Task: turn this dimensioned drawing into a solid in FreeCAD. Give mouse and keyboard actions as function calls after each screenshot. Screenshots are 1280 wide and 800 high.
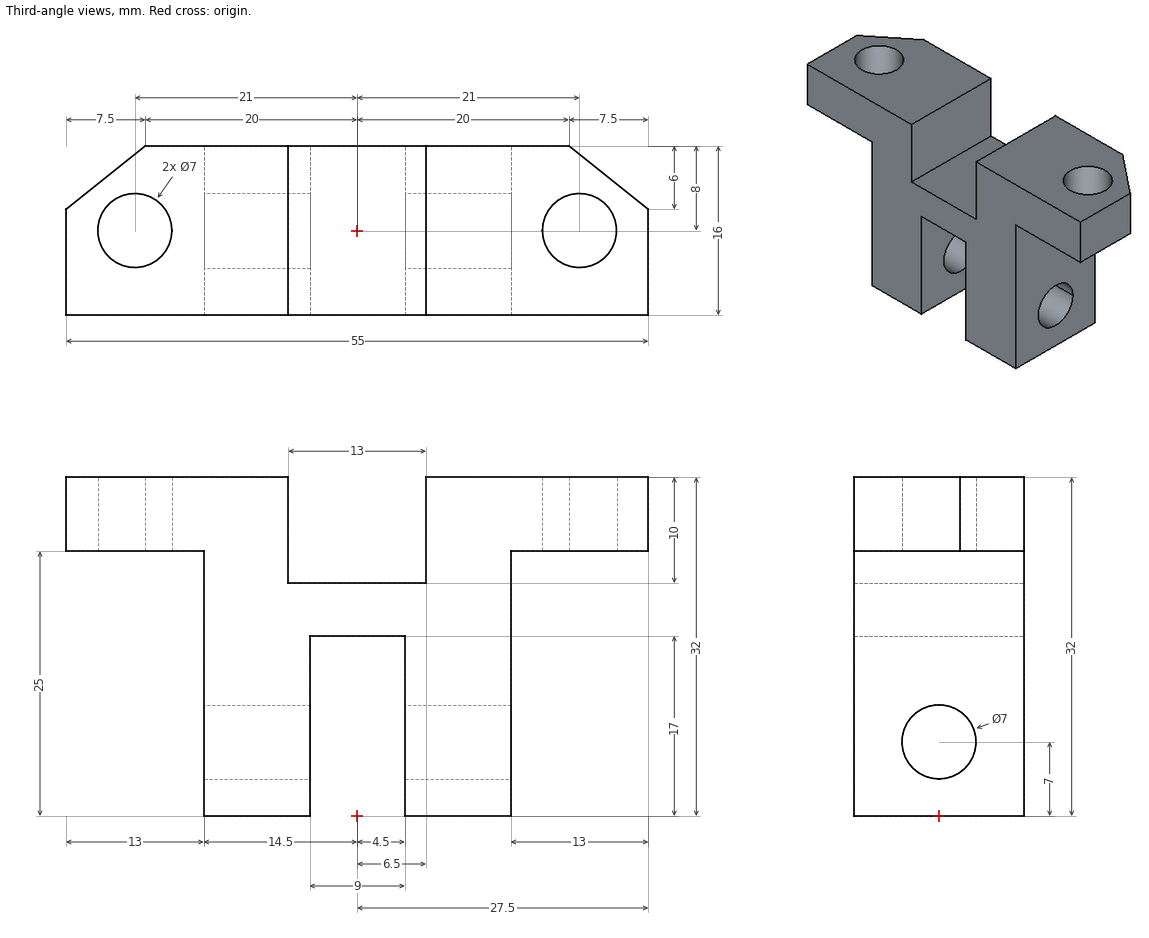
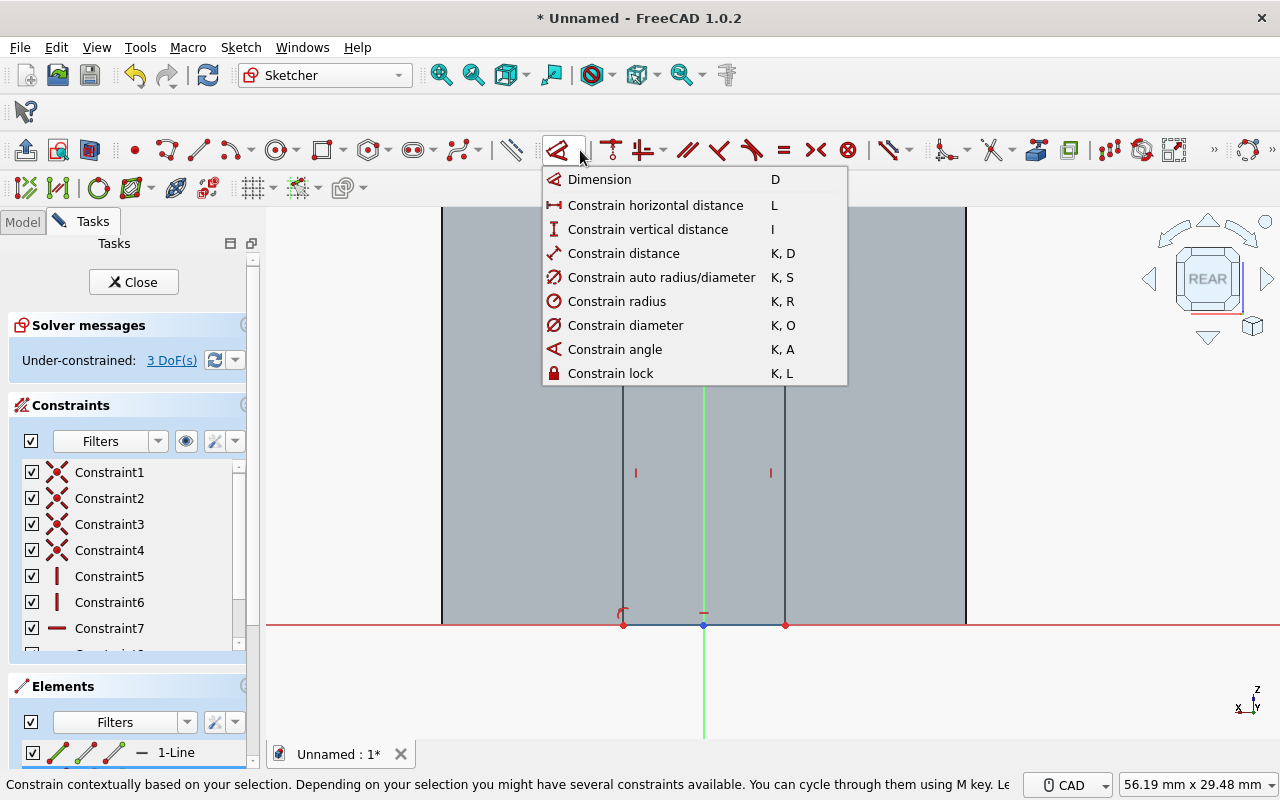
click(695, 205)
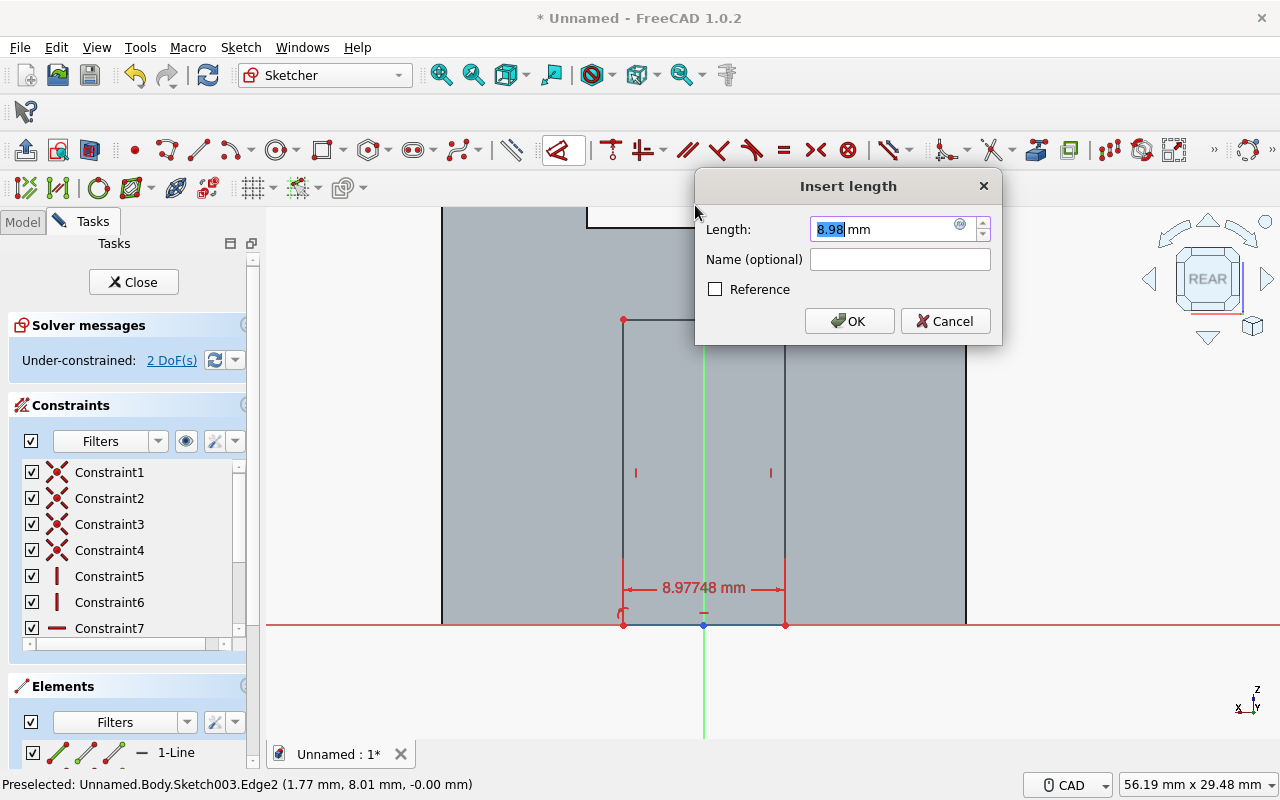
text(9)
key(Return)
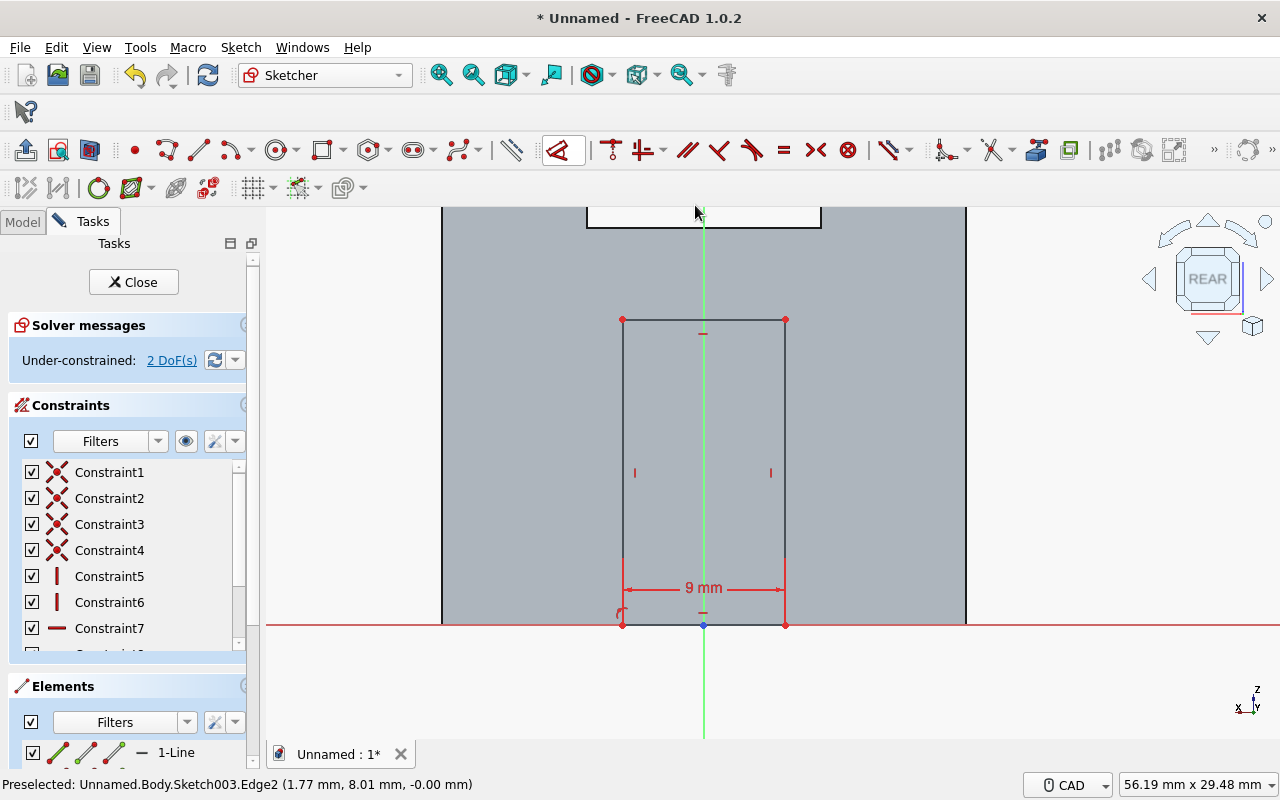
click(623, 412)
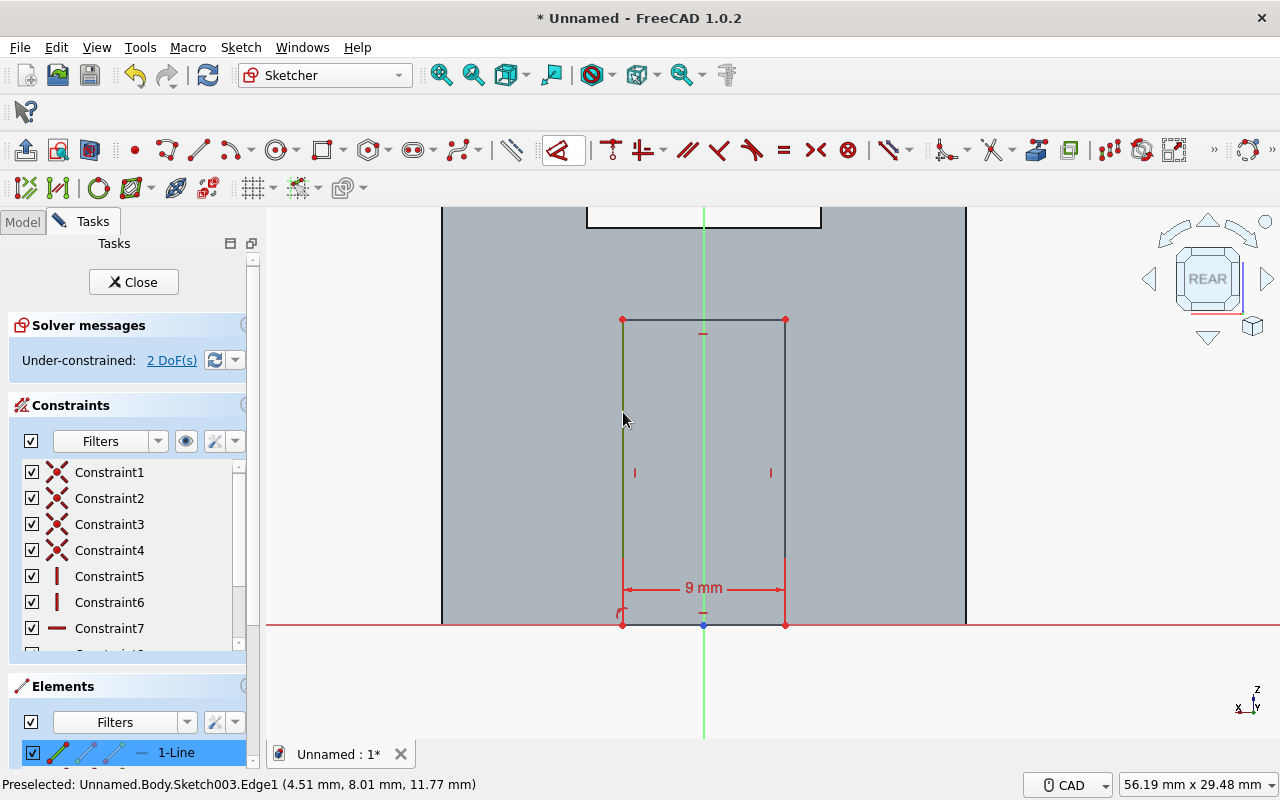
key(i)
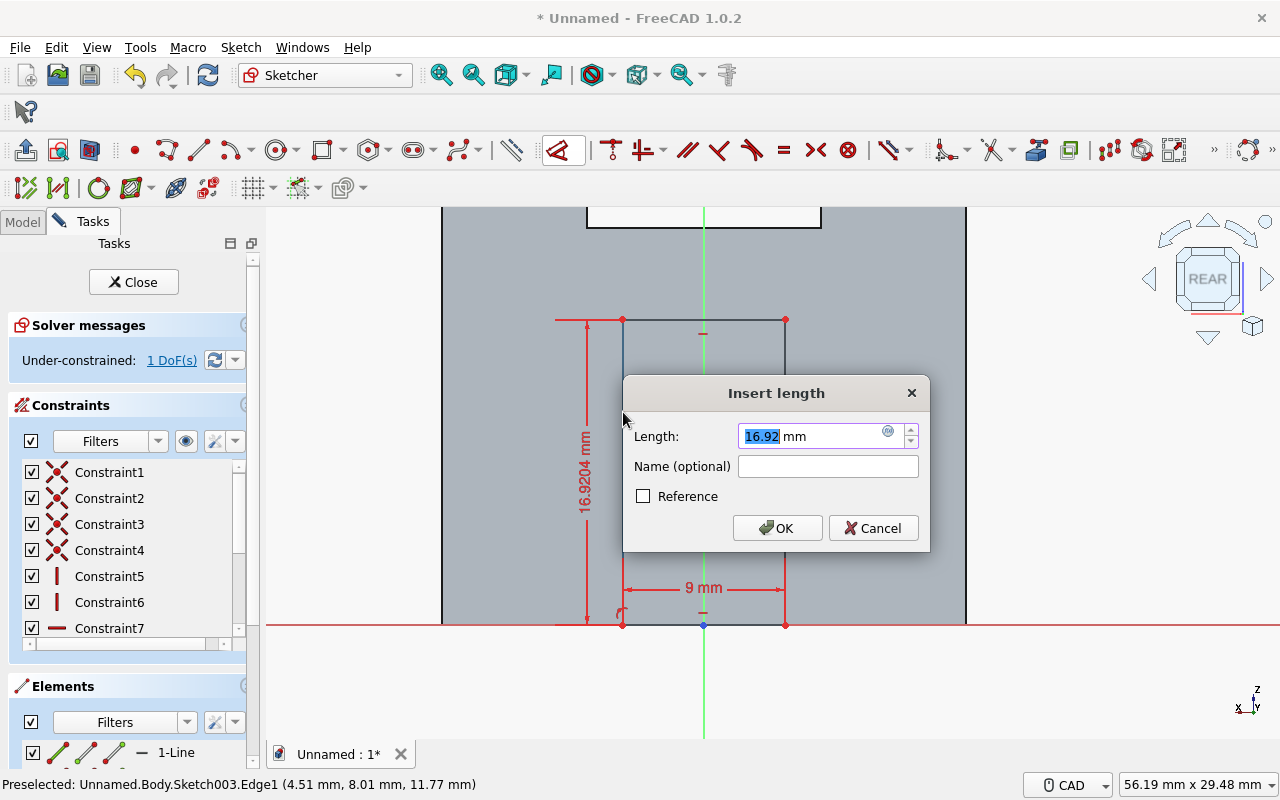
text(17)
key(Return)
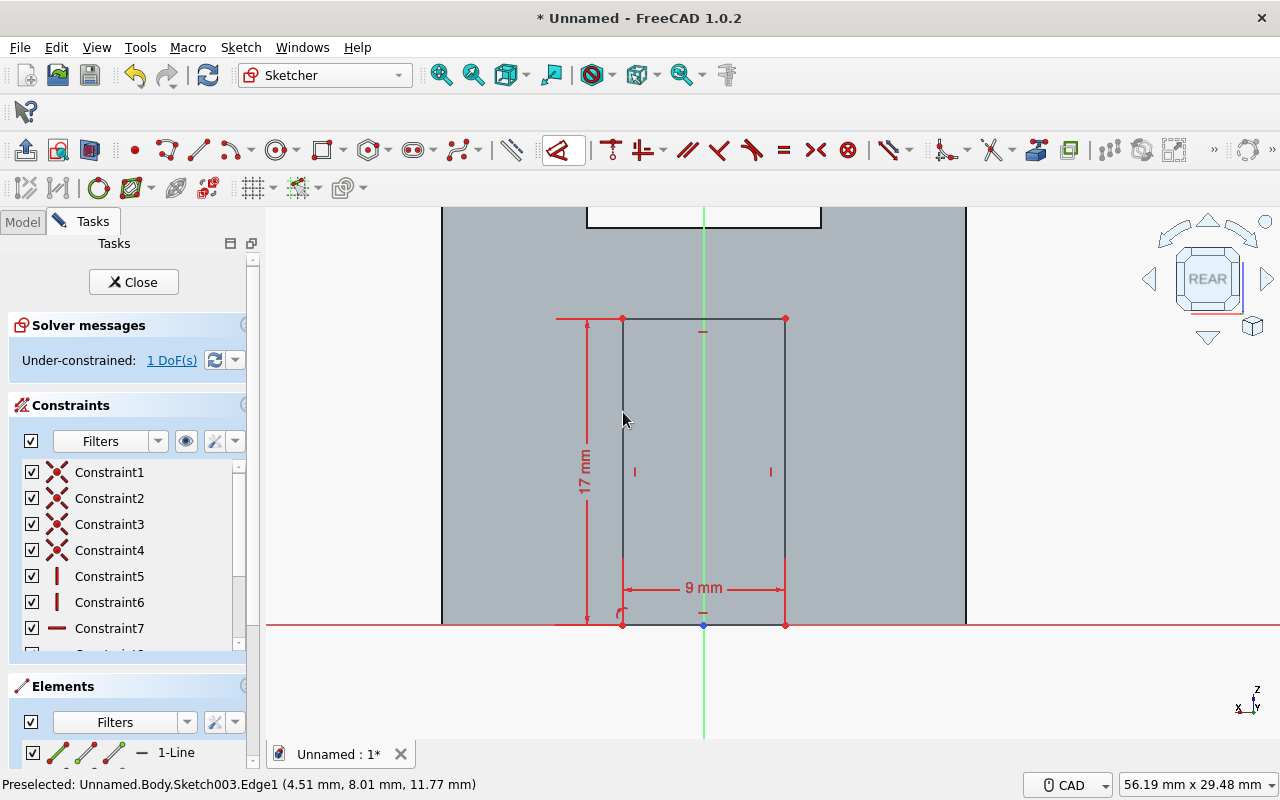
click(623, 319)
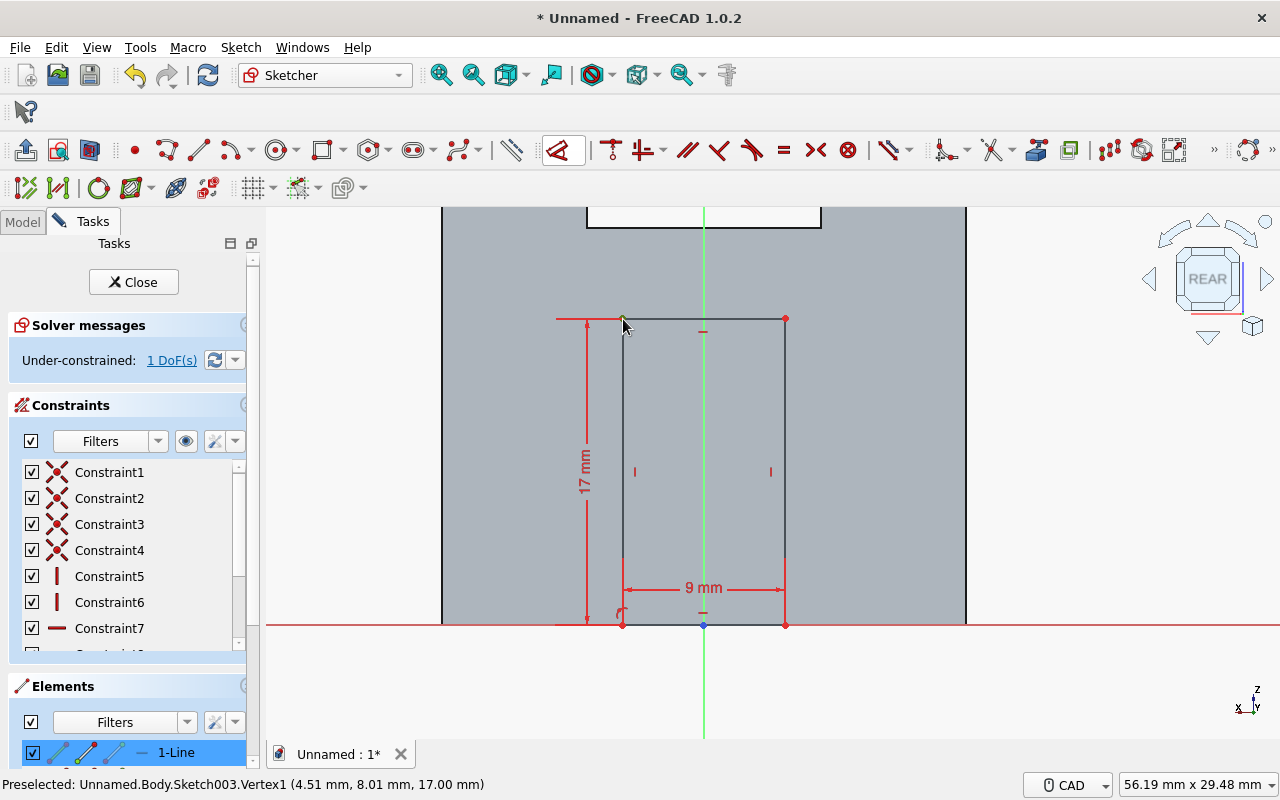
key(l)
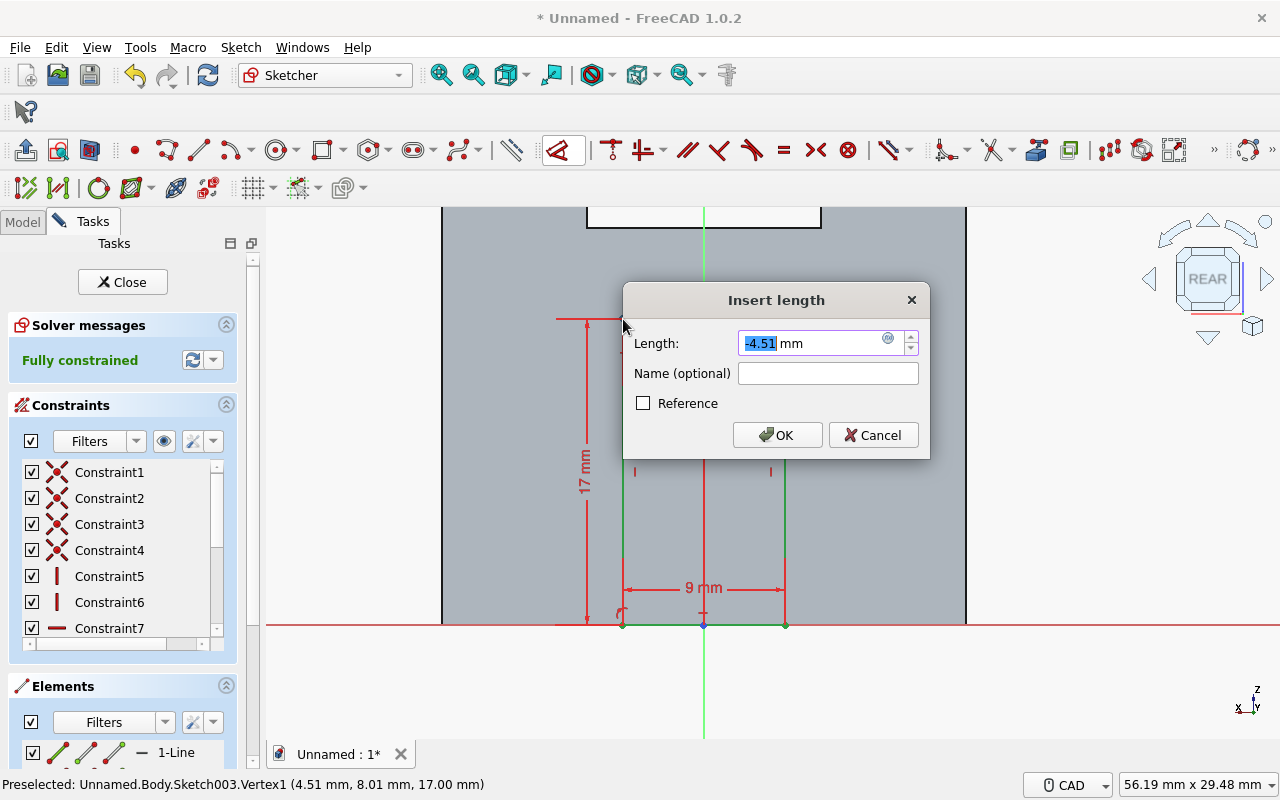
text(-4.5)
key(Return)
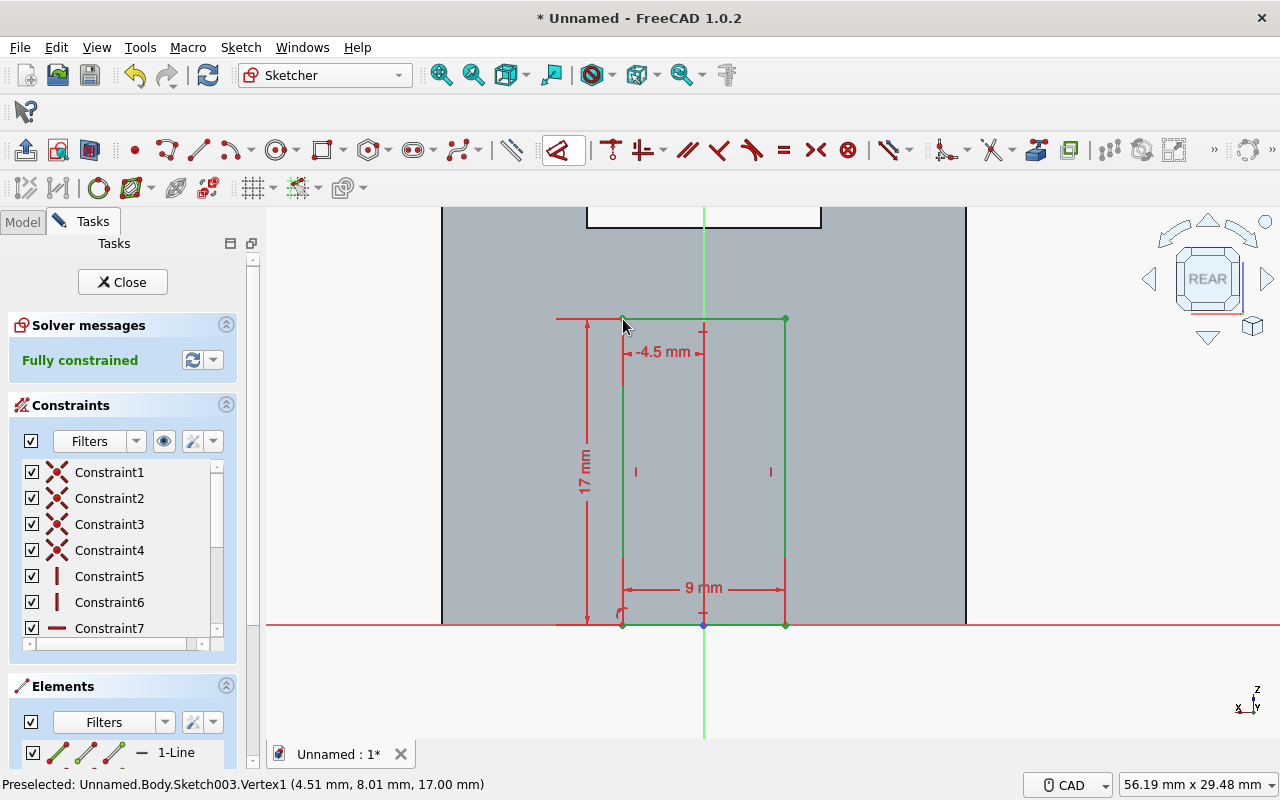
click(123, 282)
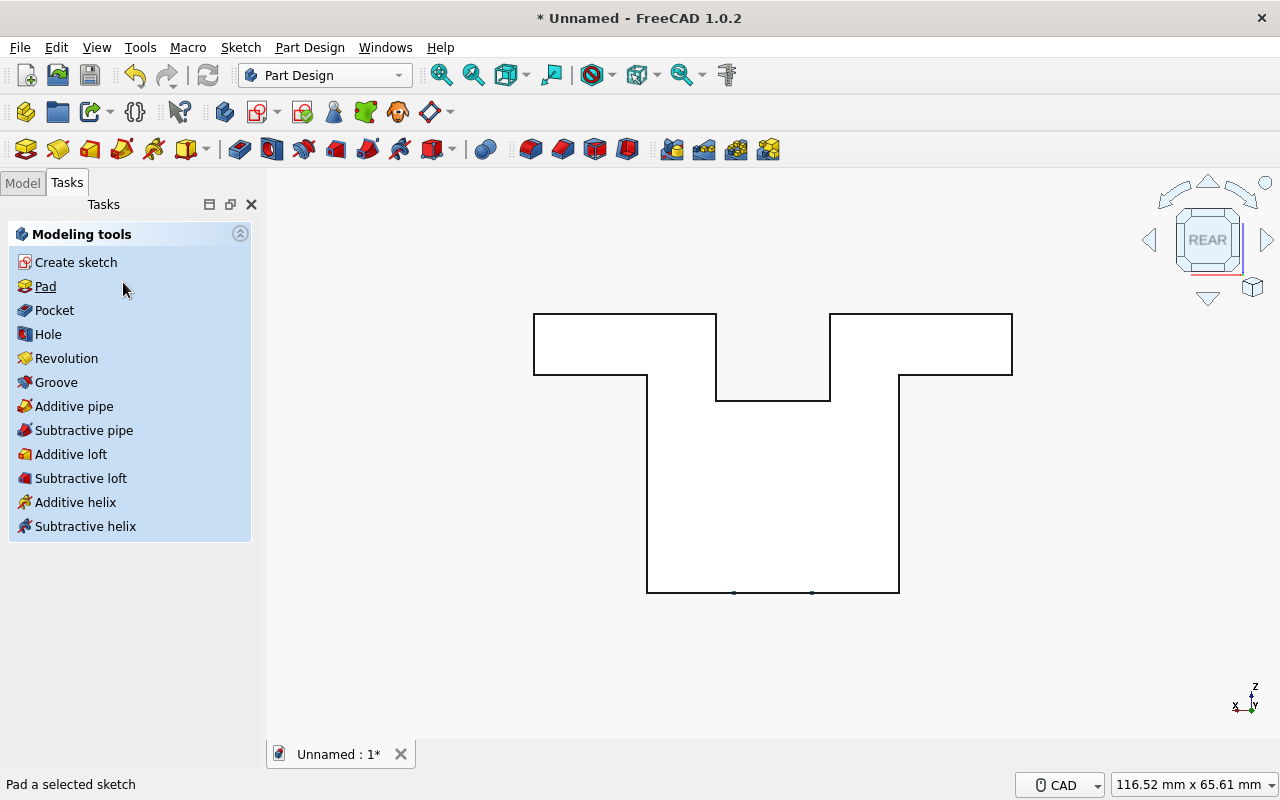
click(240, 150)